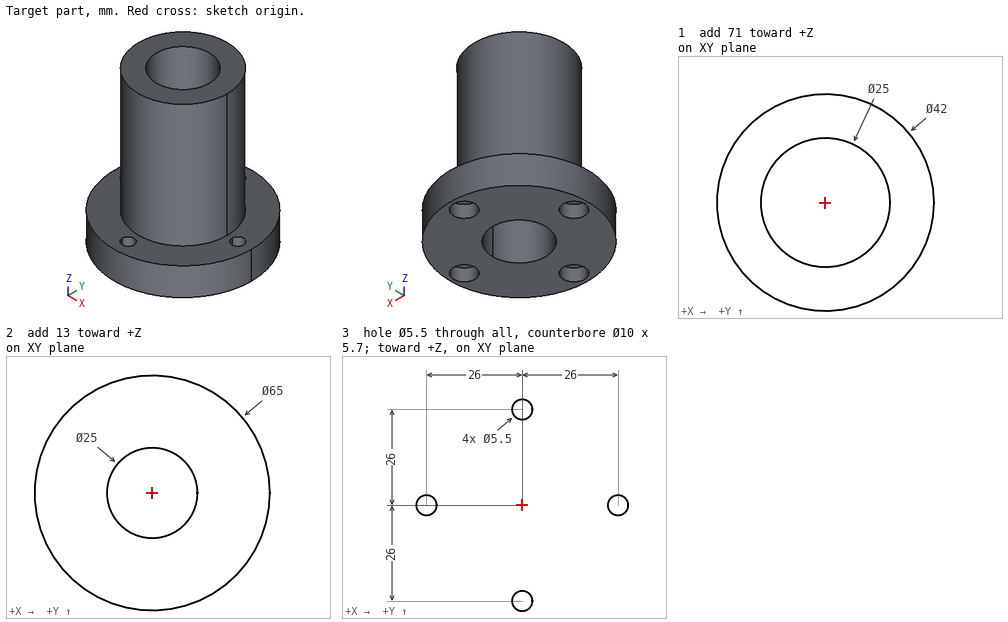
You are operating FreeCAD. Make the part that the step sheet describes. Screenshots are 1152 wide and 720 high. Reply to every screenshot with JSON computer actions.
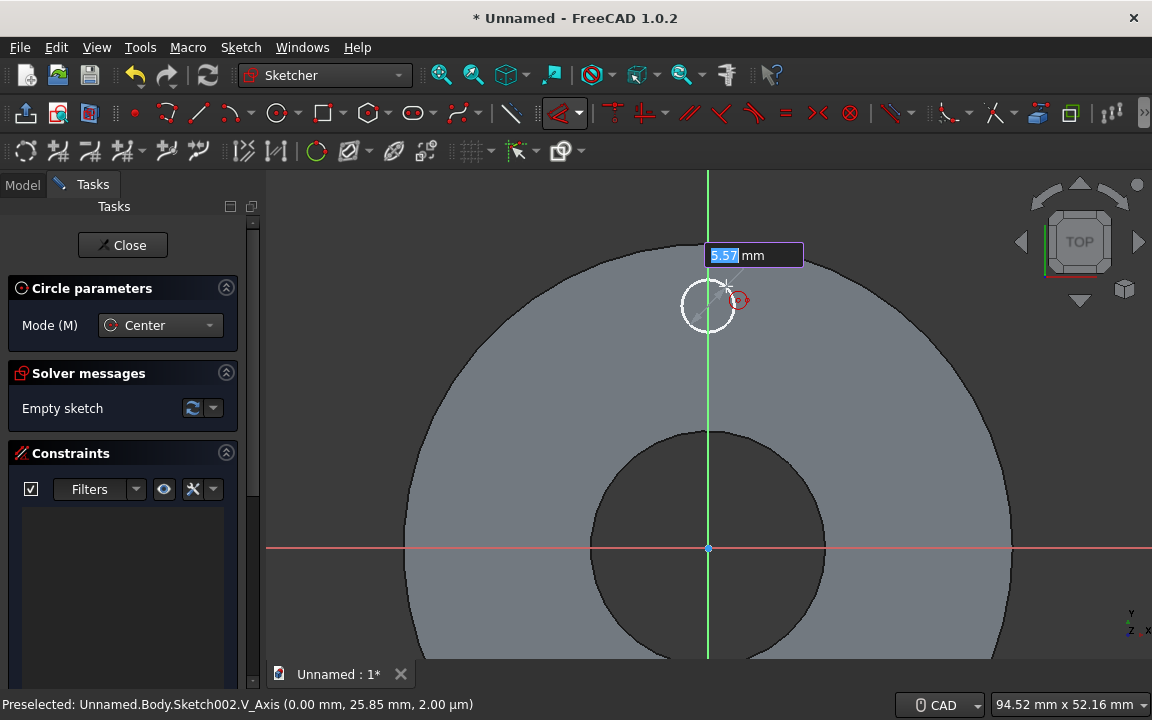
{"action": "type", "text": "5.5"}
{"action": "key", "text": "Return"}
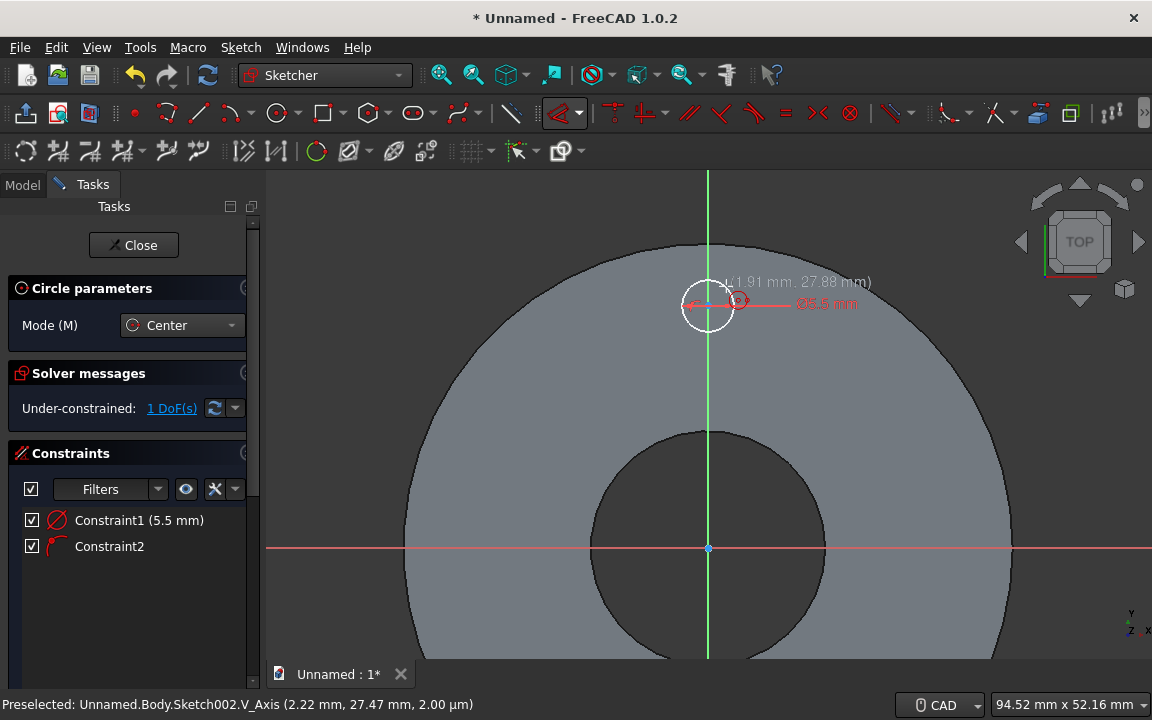
{"action": "left_click", "coordinate": [464, 548]}
{"action": "mouse_move", "coordinate": [483, 530]}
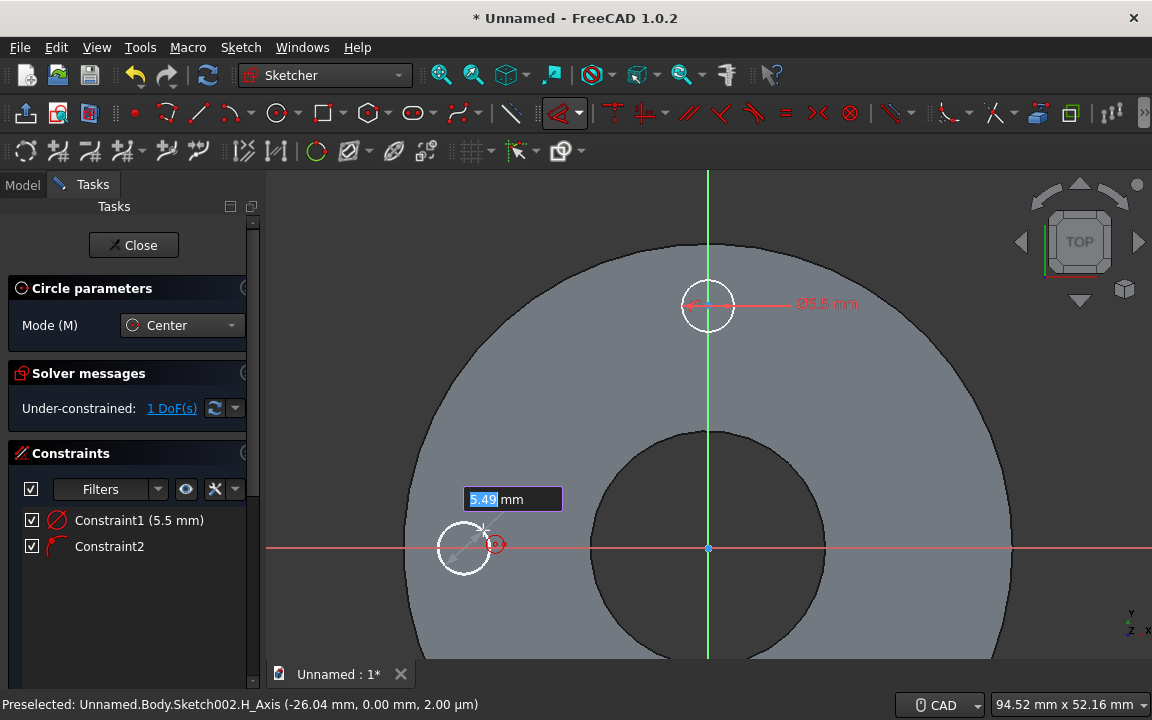
{"action": "type", "text": "5.5"}
{"action": "key", "text": "Return"}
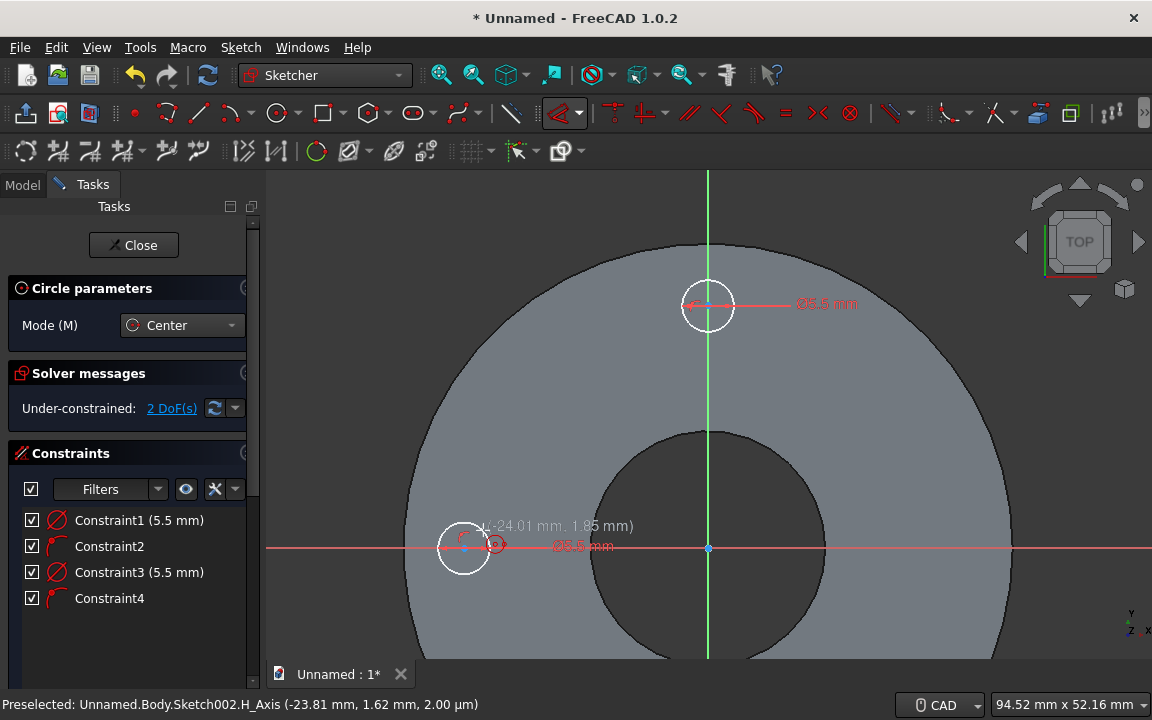
{"action": "scroll", "coordinate": [558, 252], "scroll_direction": "down", "scroll_amount": 3}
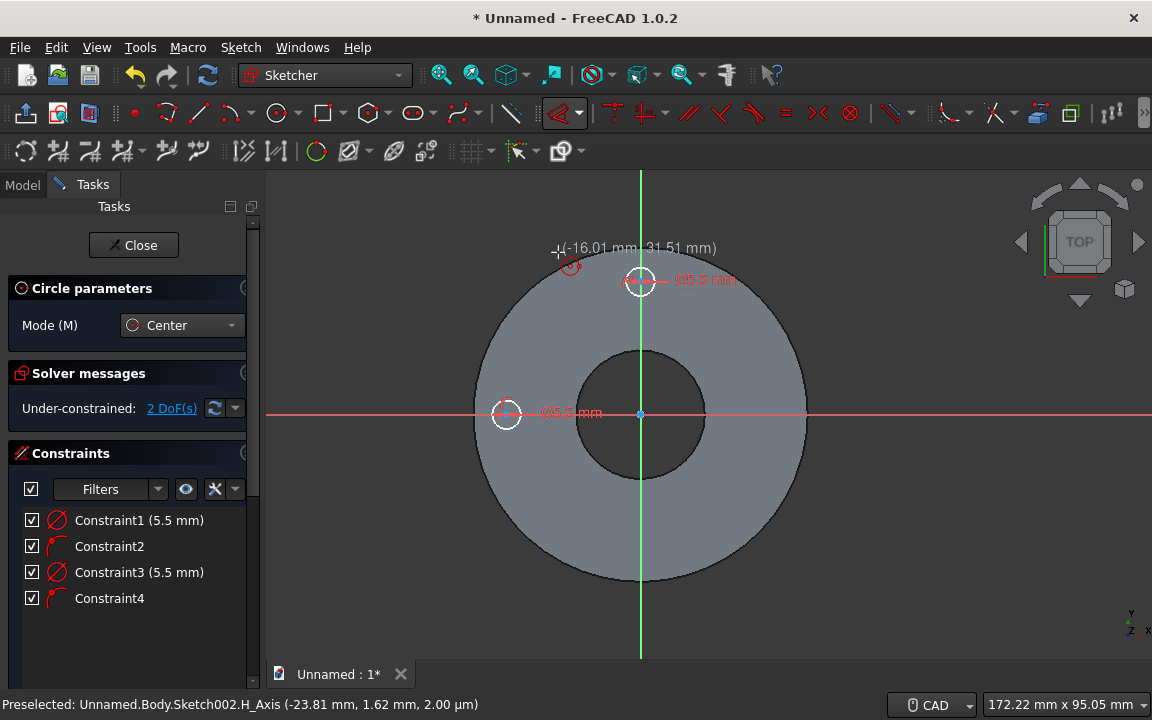
{"action": "scroll", "coordinate": [641, 548], "scroll_direction": "up", "scroll_amount": 3}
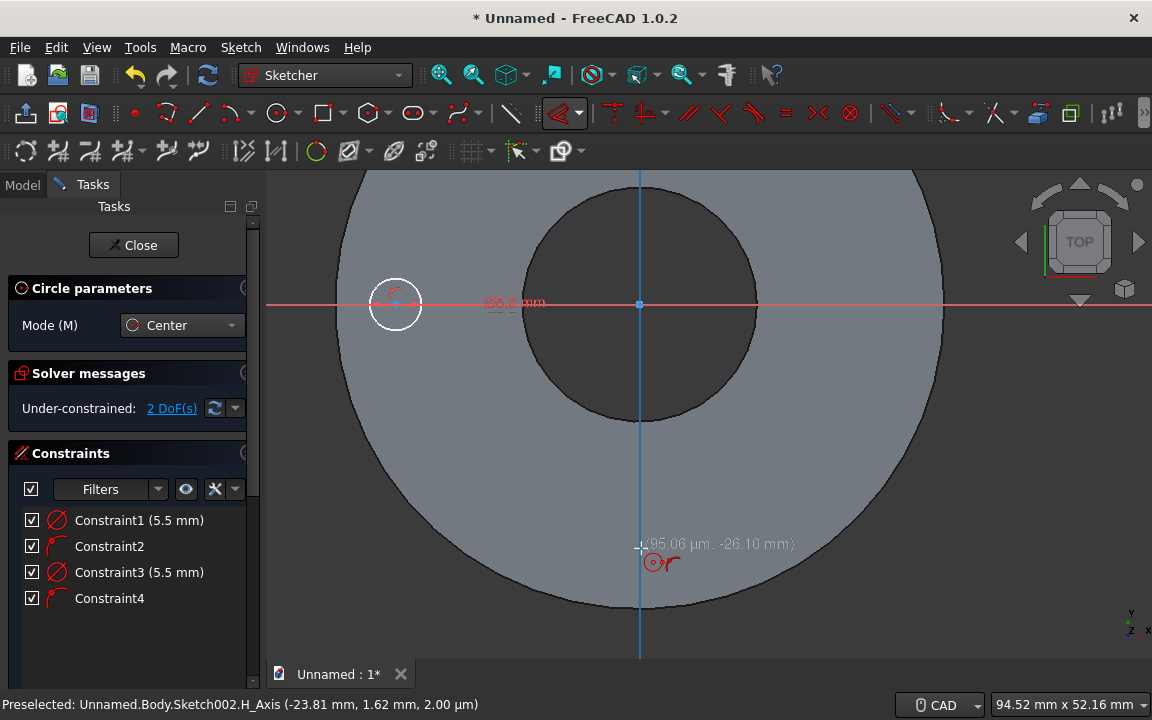
{"action": "left_click", "coordinate": [640, 548]}
{"action": "mouse_move", "coordinate": [658, 530]}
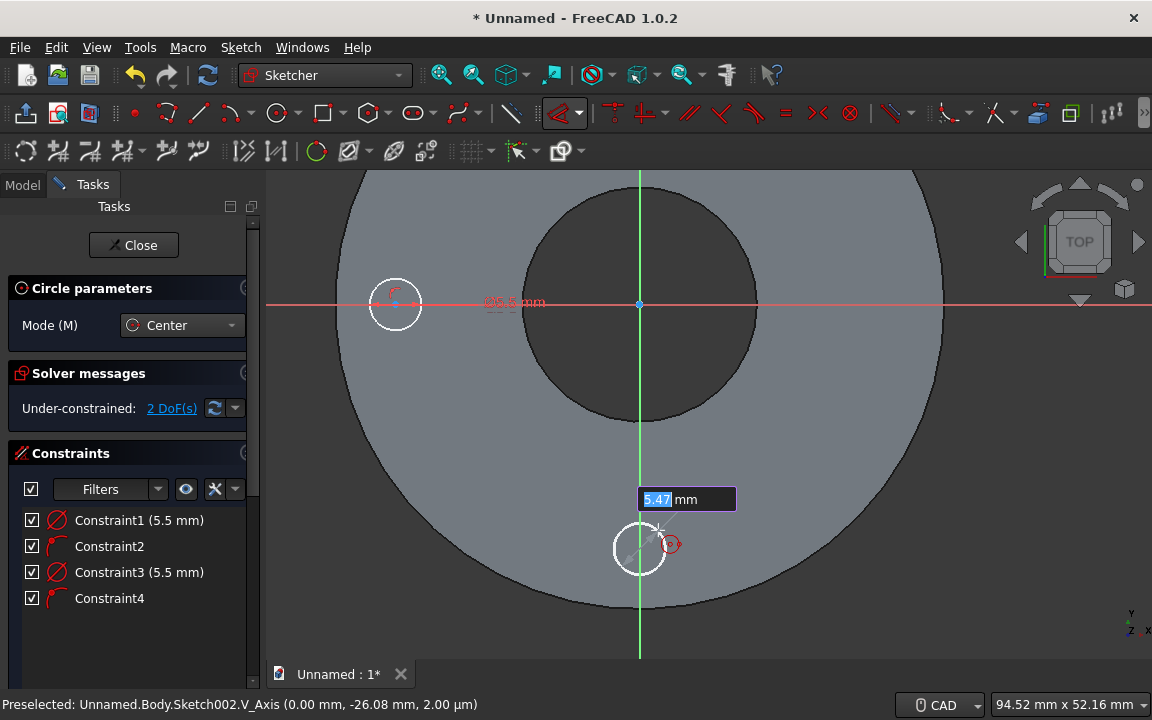
{"action": "type", "text": "5.5"}
{"action": "key", "text": "Return"}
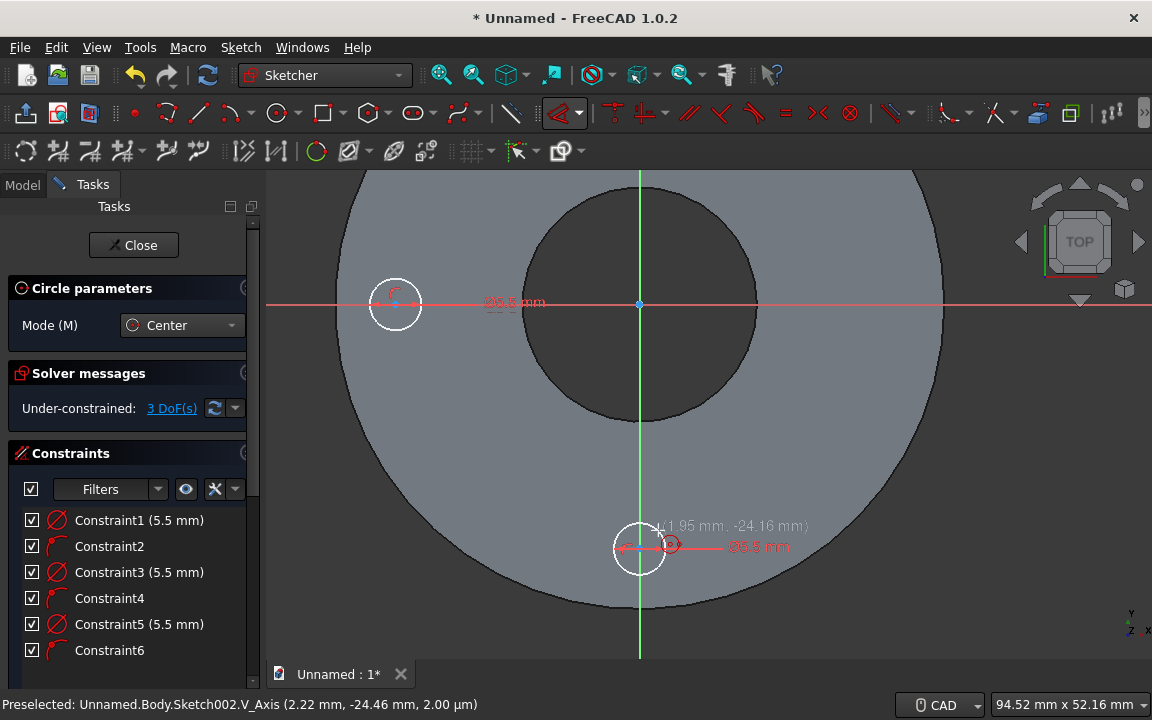
{"action": "left_click", "coordinate": [883, 305]}
{"action": "mouse_move", "coordinate": [902, 286]}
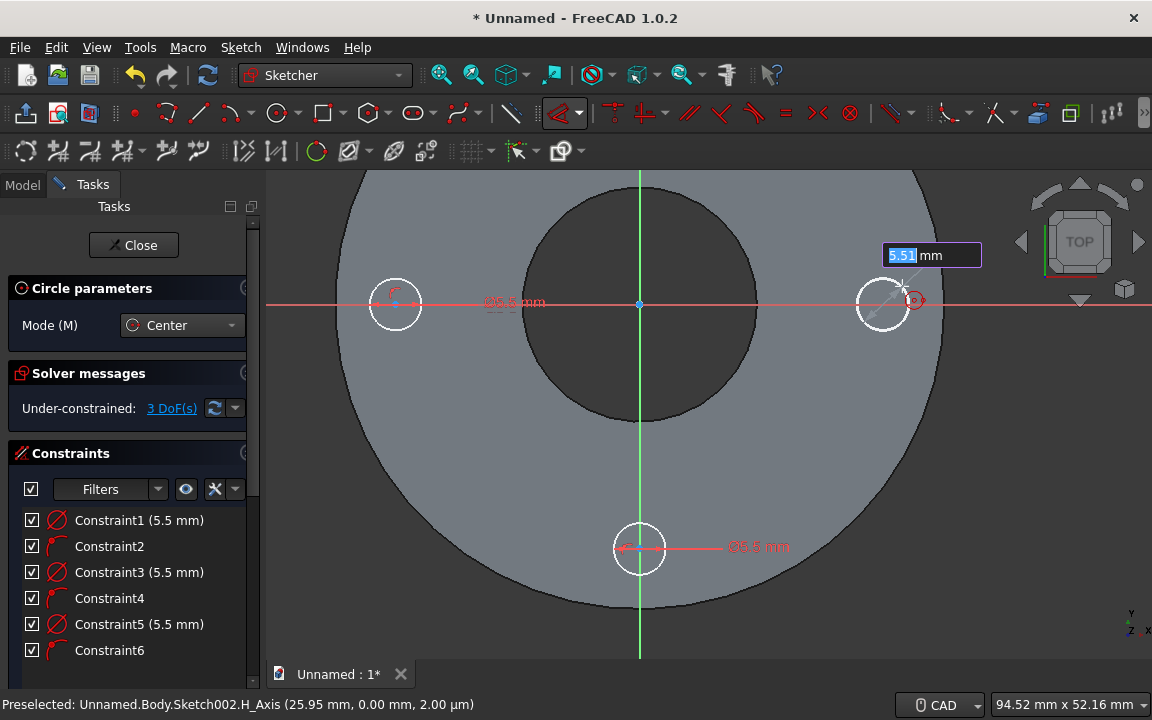
{"action": "type", "text": "5.5"}
{"action": "key", "text": "Return"}
{"action": "key", "text": "Escape"}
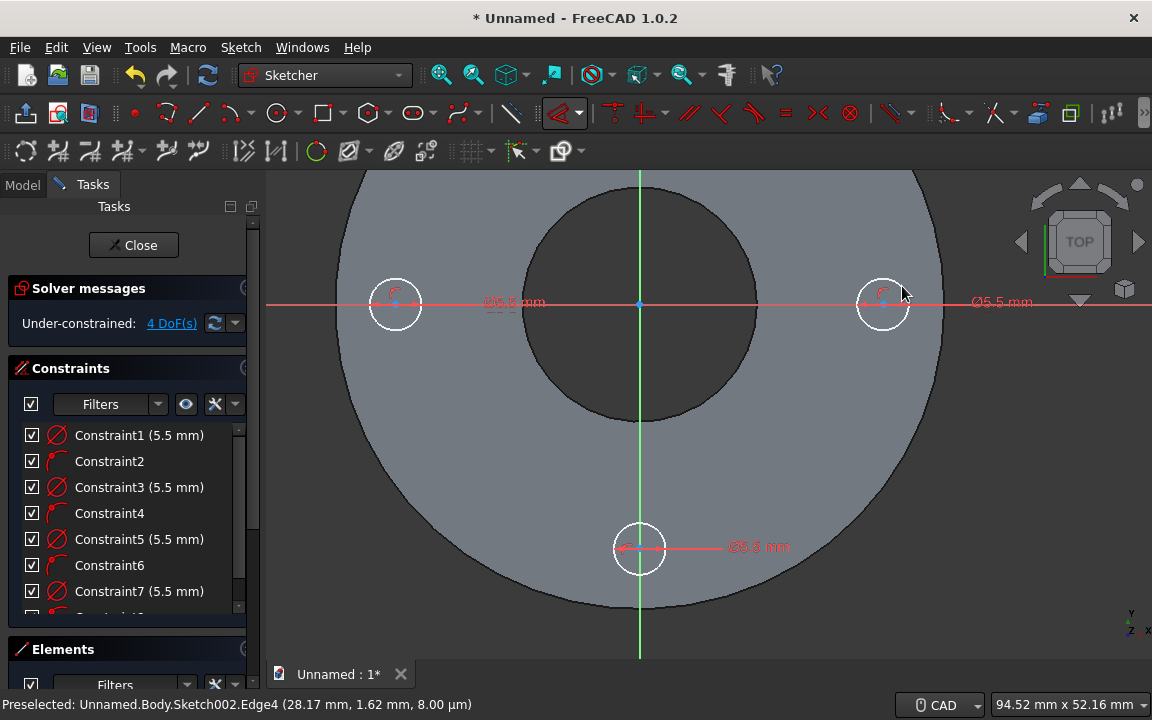
{"action": "left_click", "coordinate": [558, 114]}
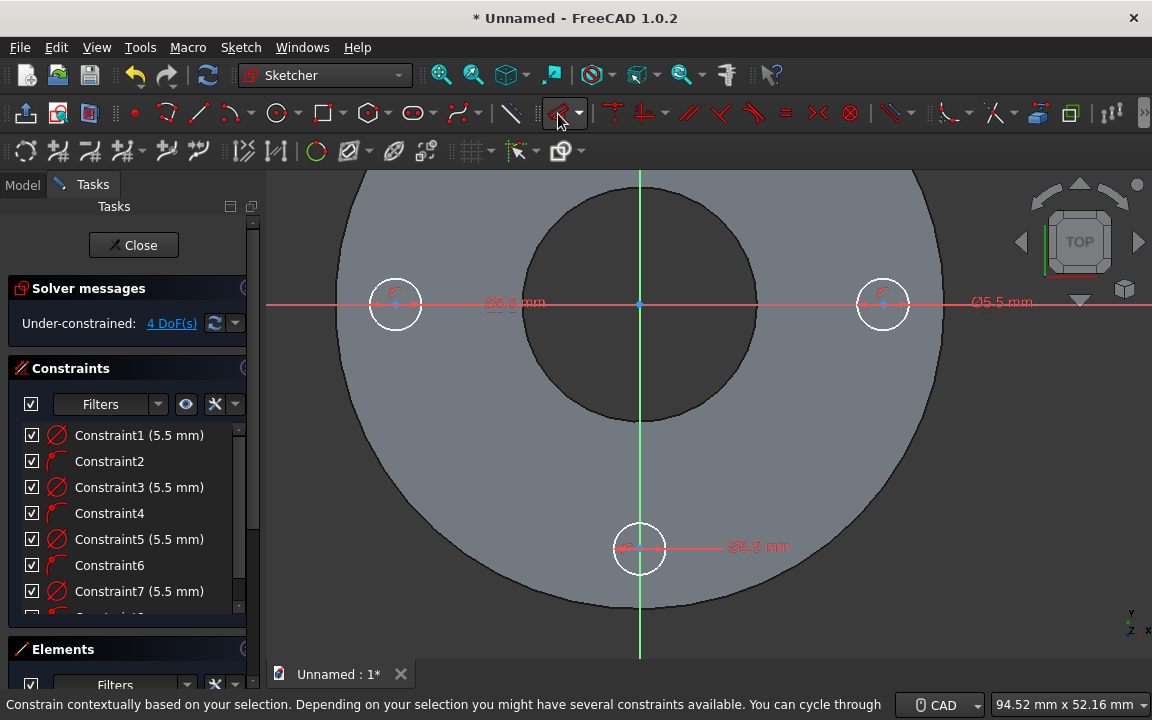
{"action": "scroll", "coordinate": [641, 548], "scroll_direction": "down", "scroll_amount": 3}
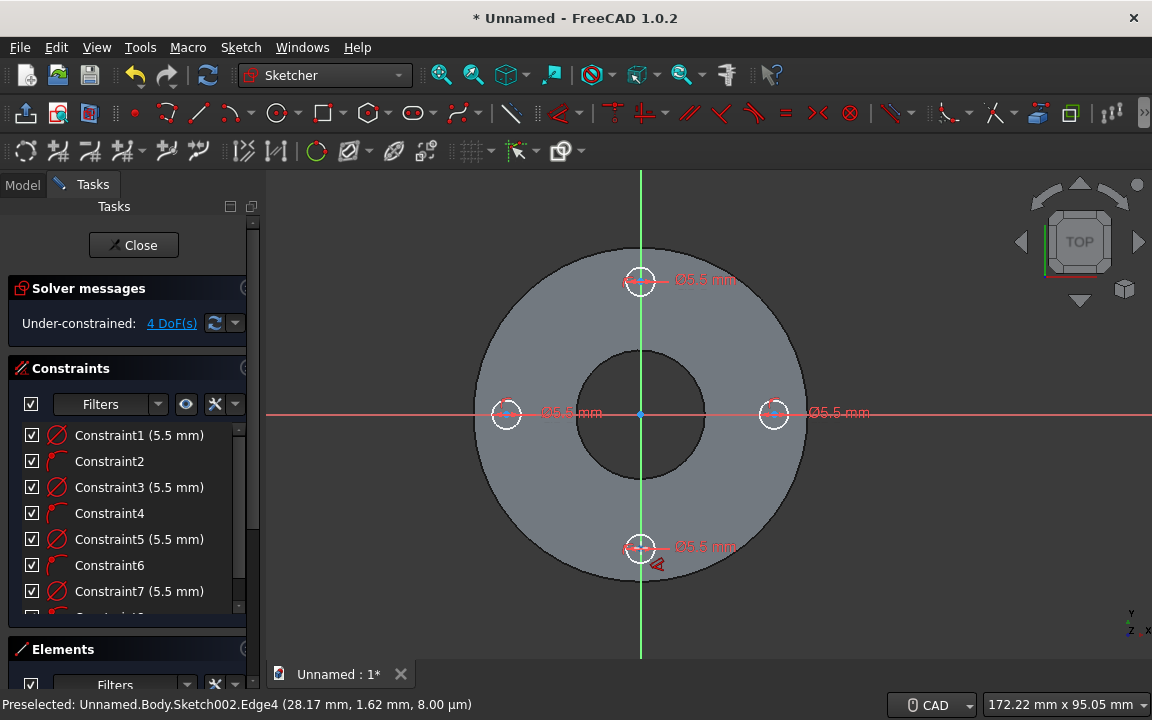
{"action": "left_click", "coordinate": [641, 282]}
{"action": "left_click", "coordinate": [675, 348]}